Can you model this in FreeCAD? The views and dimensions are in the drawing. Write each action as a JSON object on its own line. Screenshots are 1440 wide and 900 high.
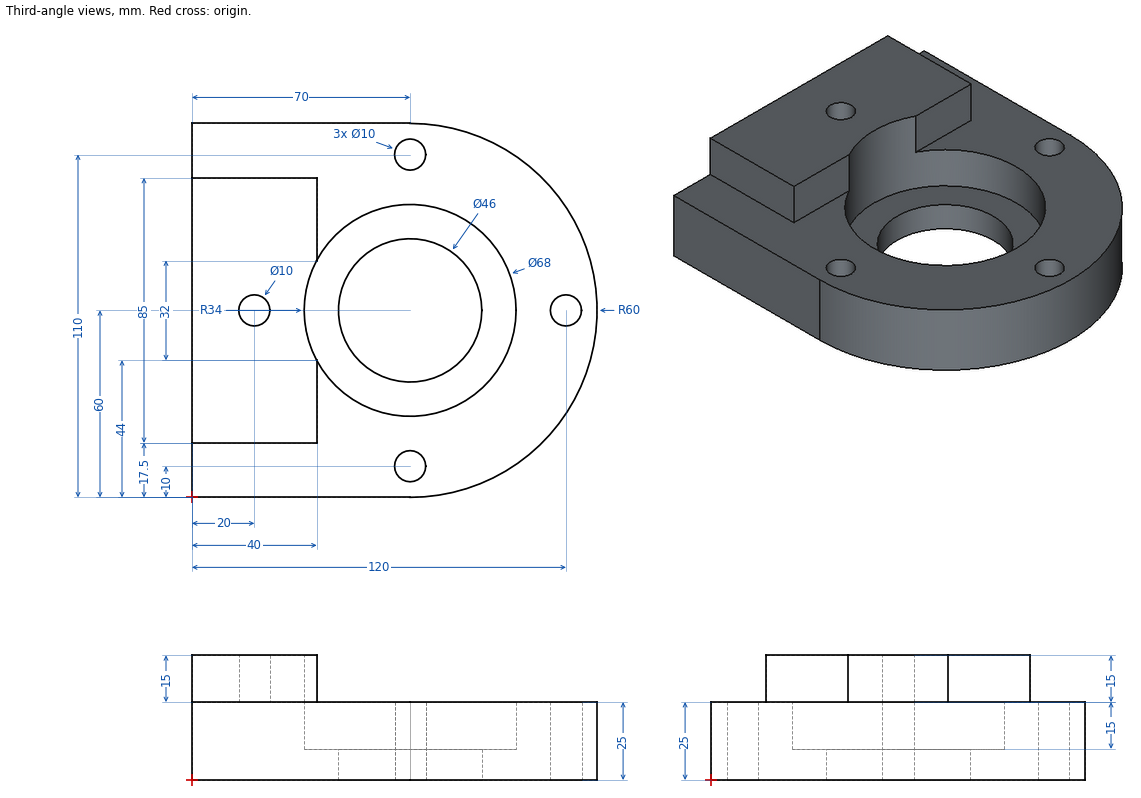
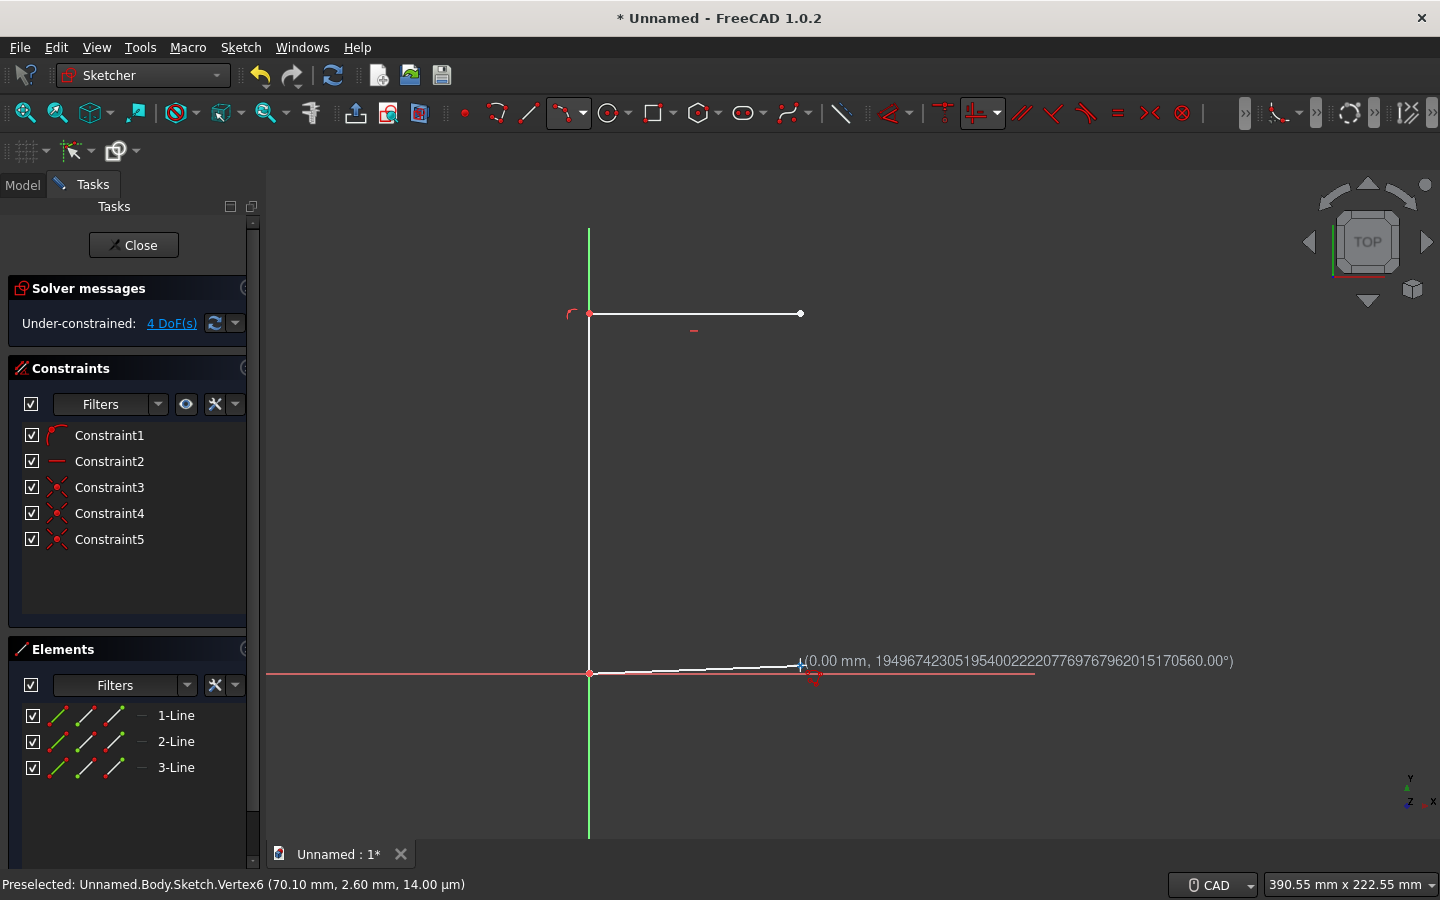
{"action": "left_click", "coordinate": [562, 114]}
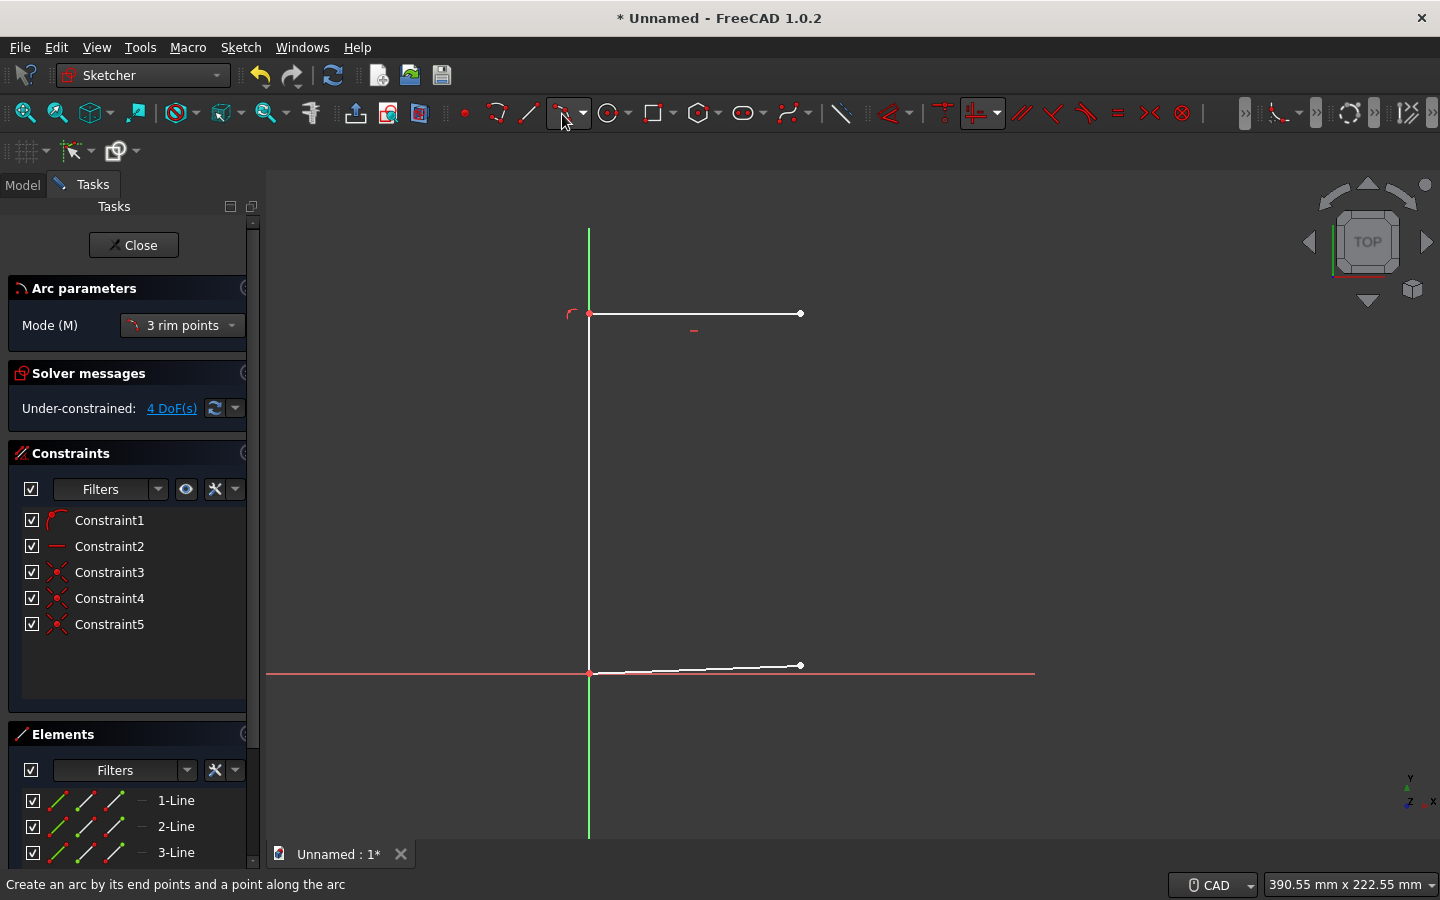
{"action": "left_click", "coordinate": [800, 666]}
{"action": "left_click", "coordinate": [800, 314]}
{"action": "left_click", "coordinate": [980, 493]}
{"action": "key", "text": "Escape"}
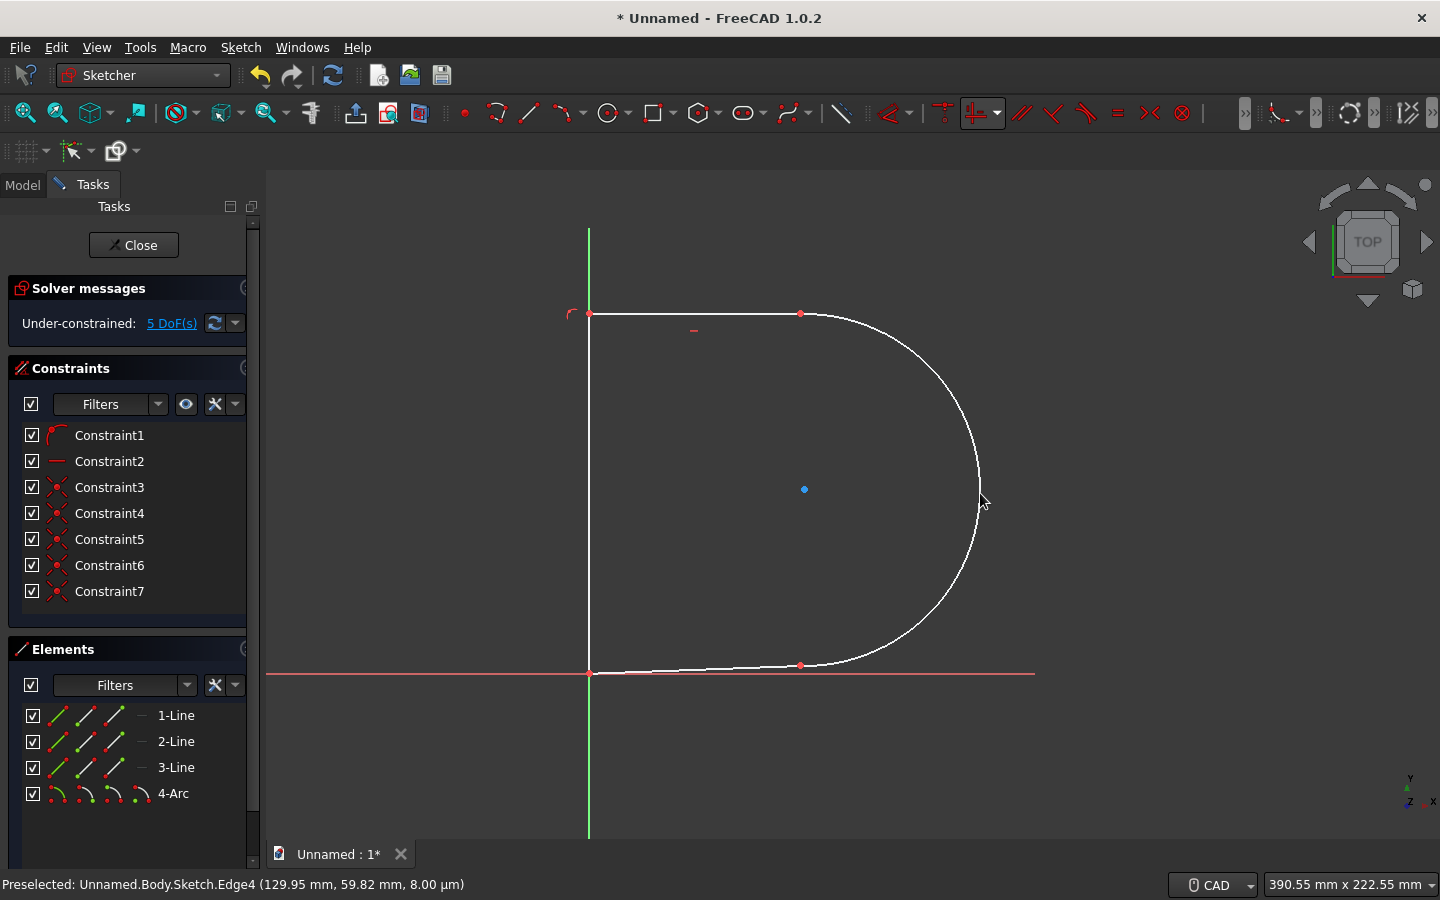
{"action": "left_click", "coordinate": [652, 671]}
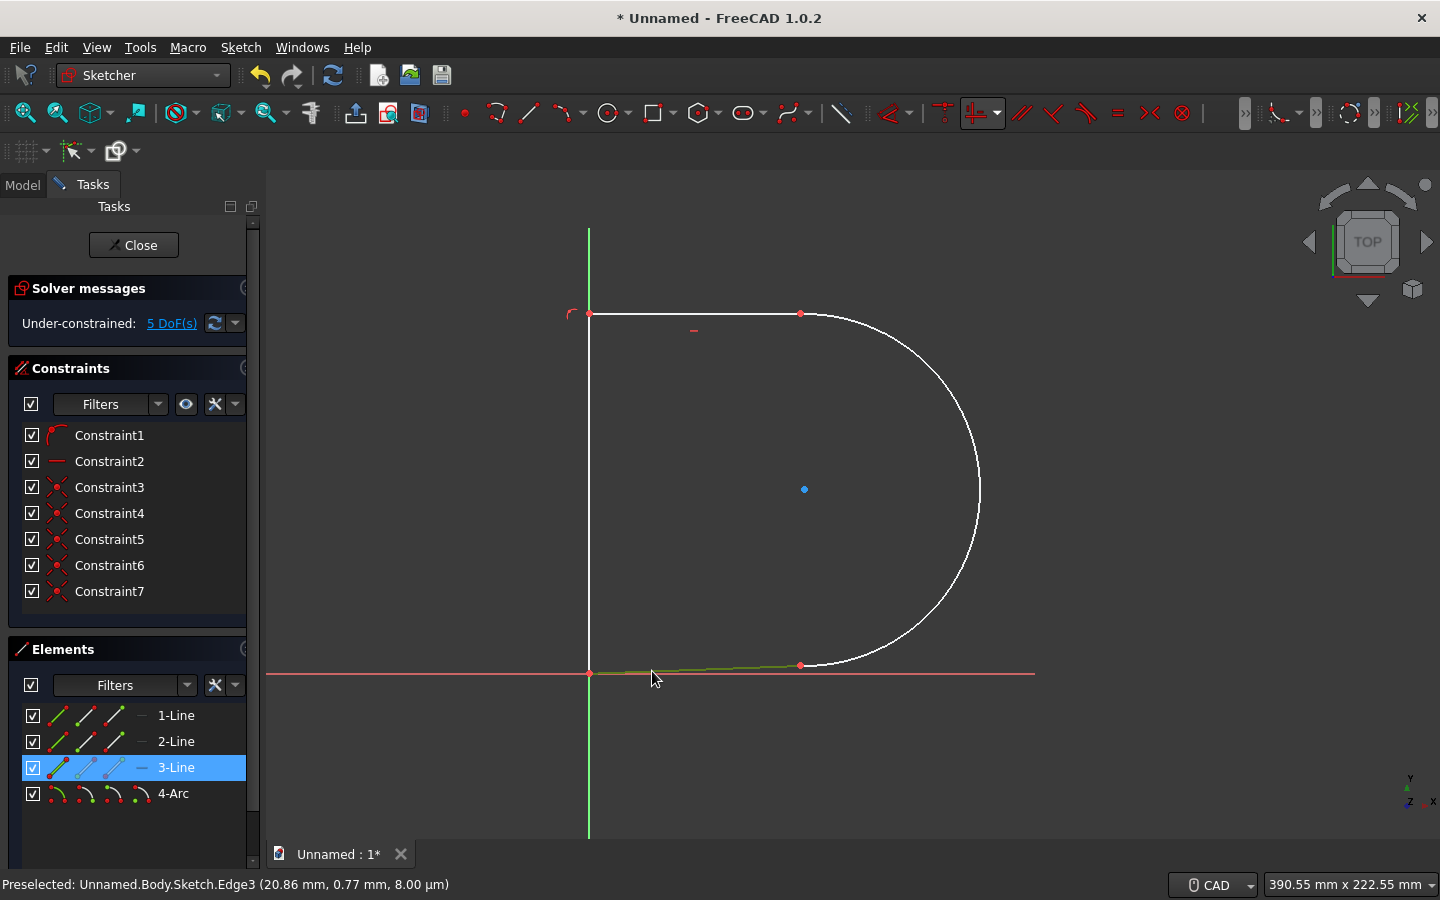
{"action": "left_click", "coordinate": [1000, 114]}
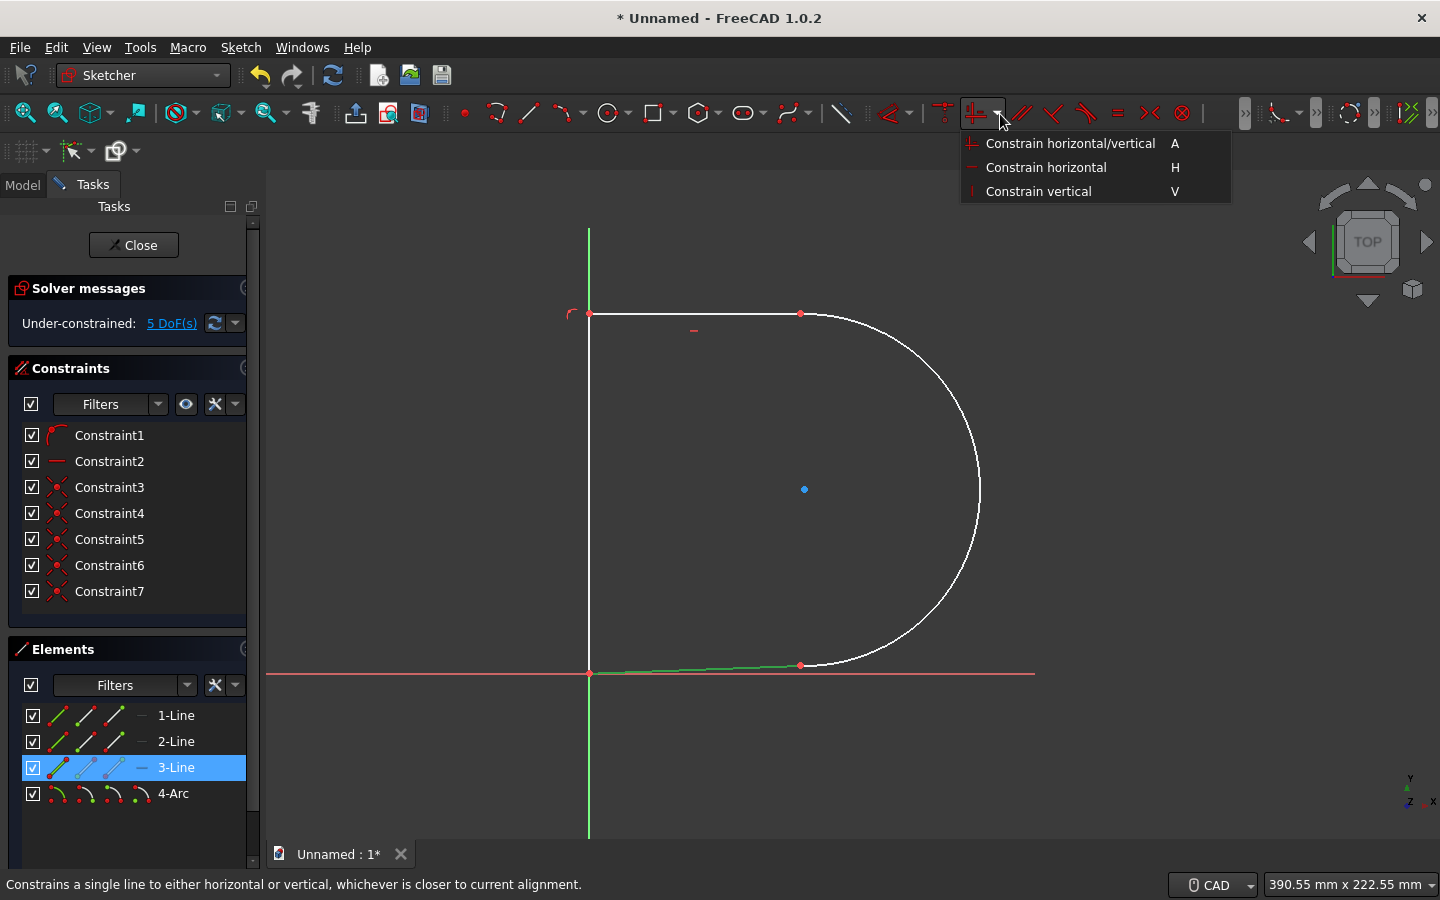
{"action": "left_click", "coordinate": [1096, 167]}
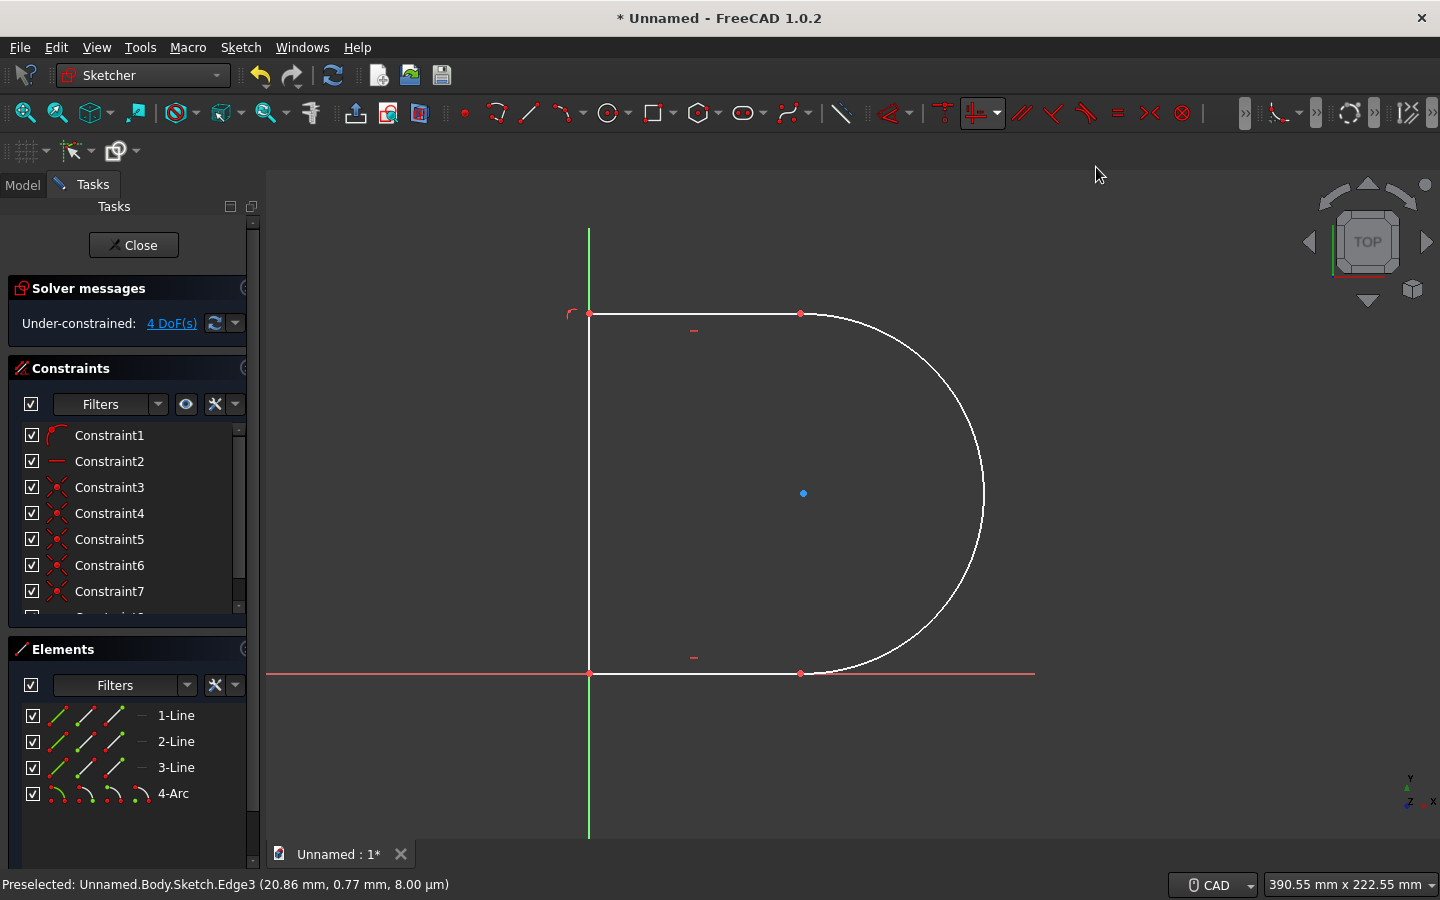
{"action": "left_click", "coordinate": [949, 601]}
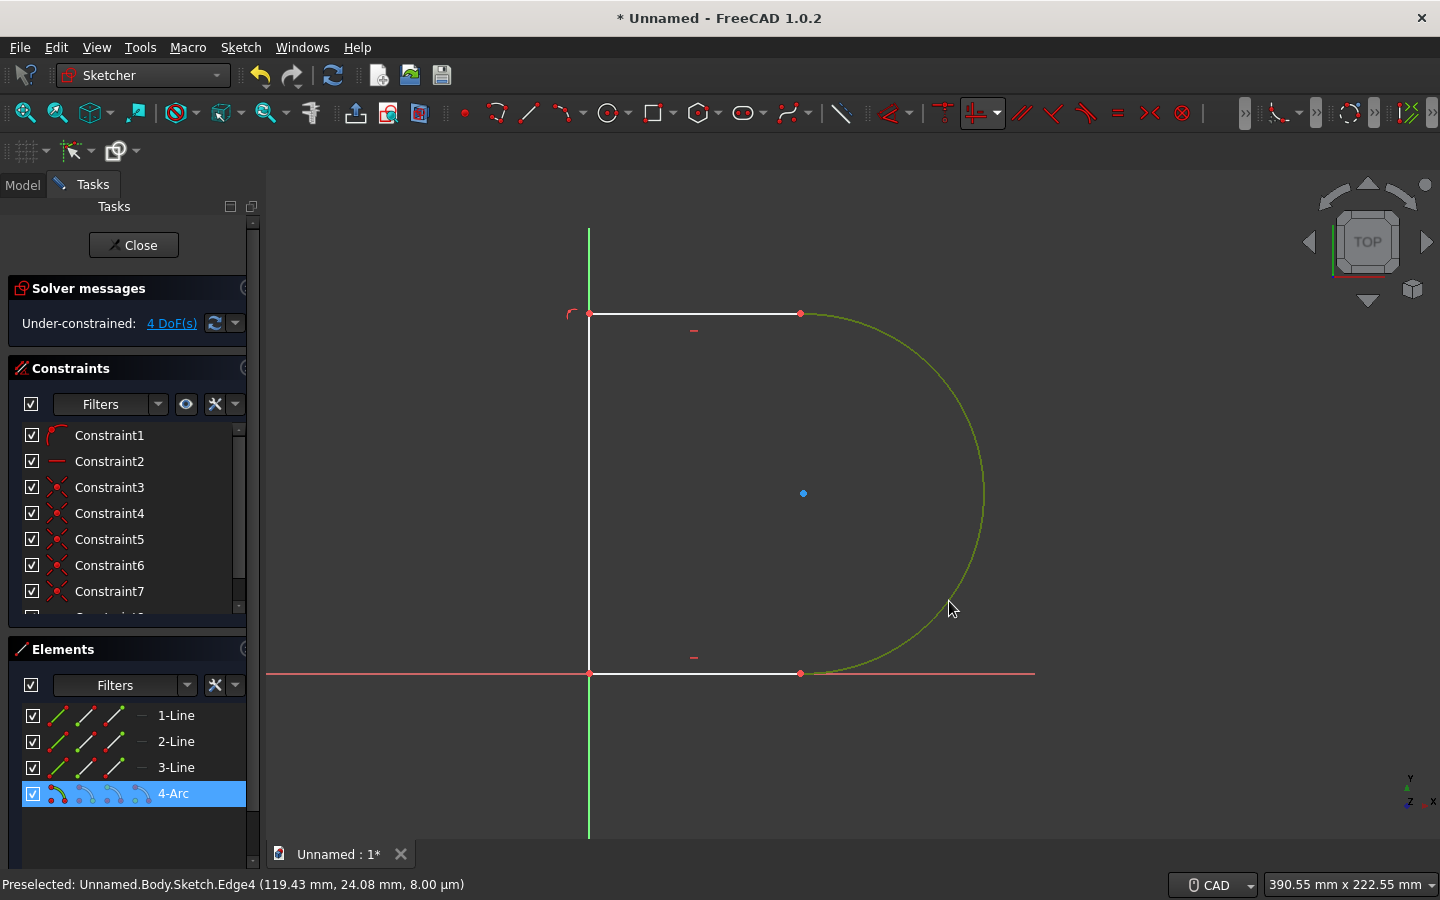
{"action": "left_click", "coordinate": [912, 114]}